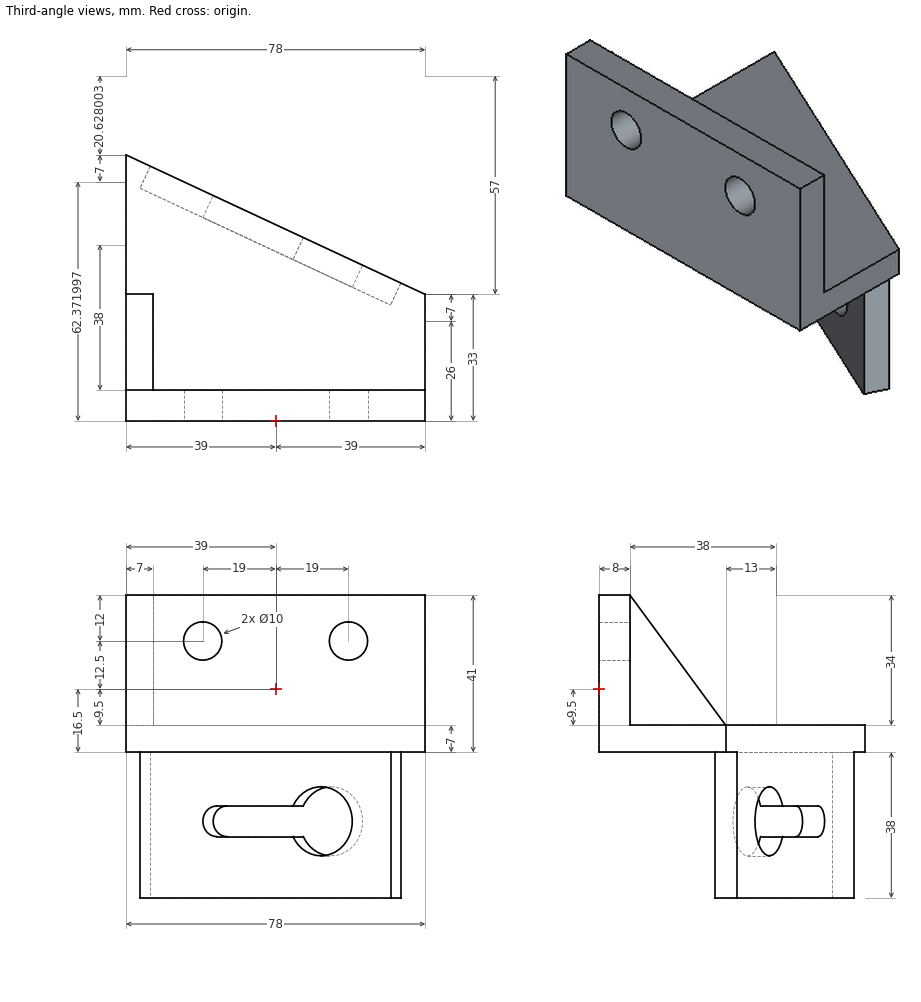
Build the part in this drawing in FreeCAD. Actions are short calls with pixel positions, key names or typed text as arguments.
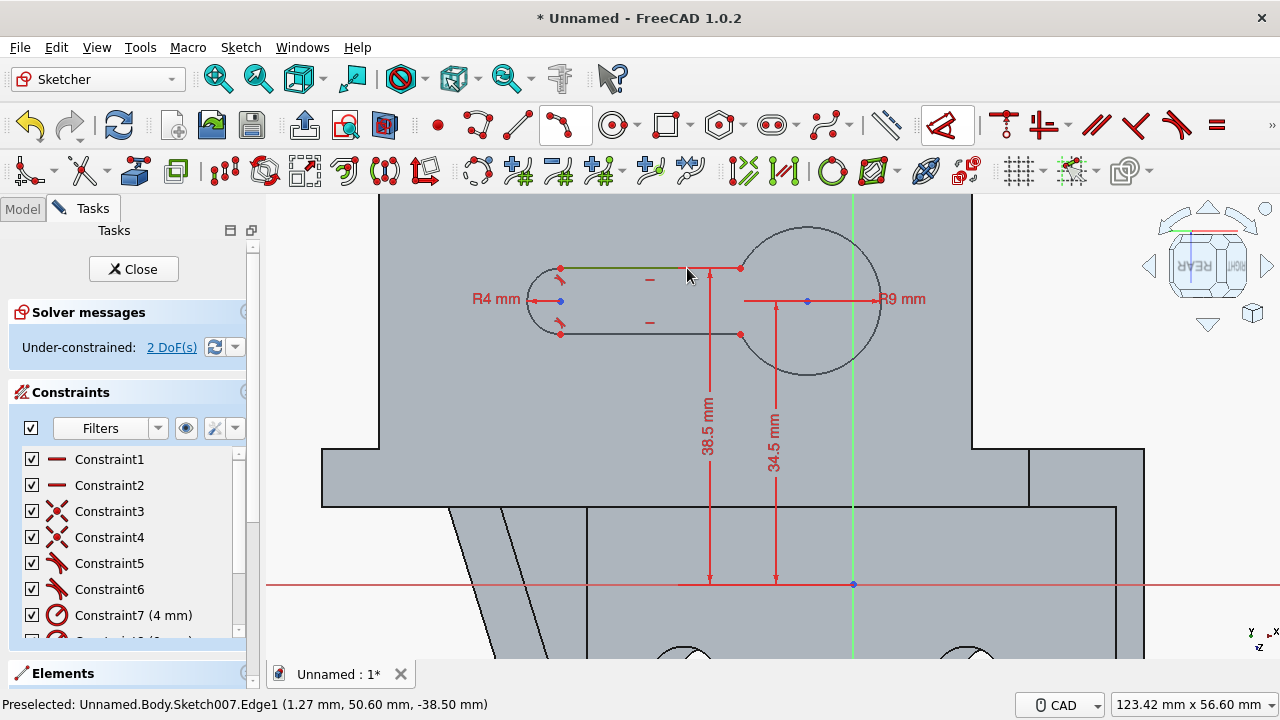
key(l)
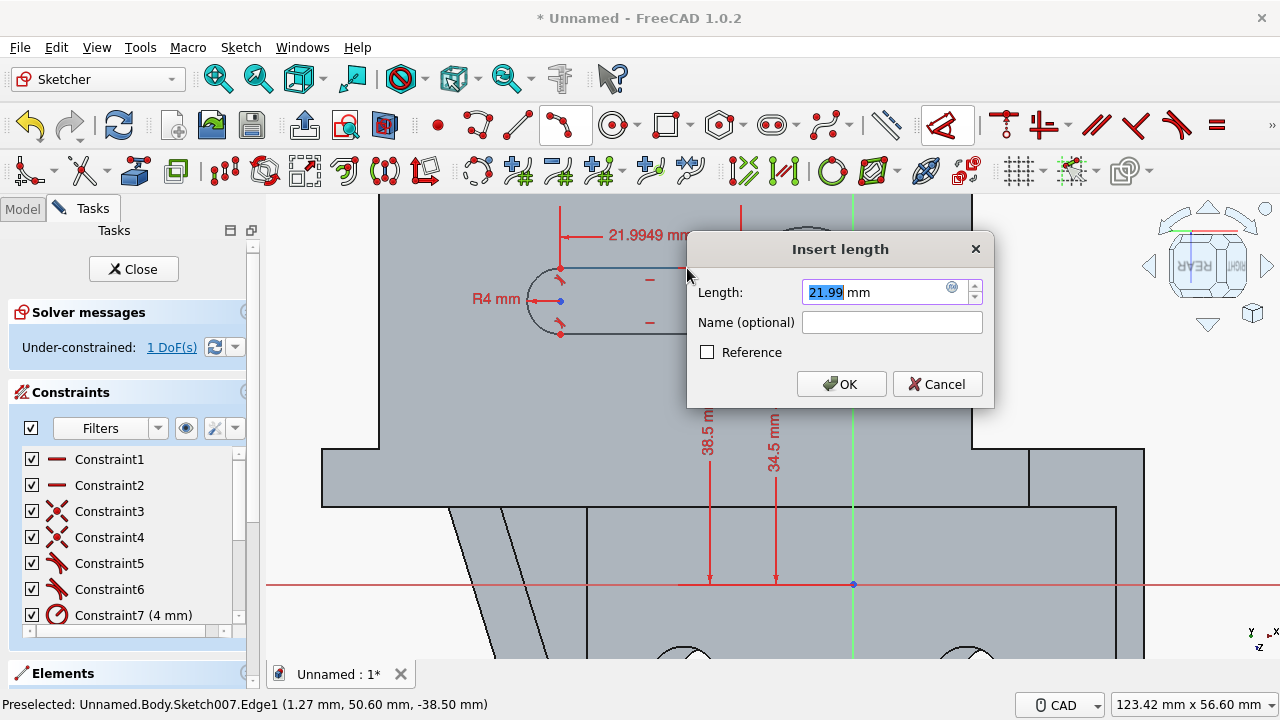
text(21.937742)
key(Return)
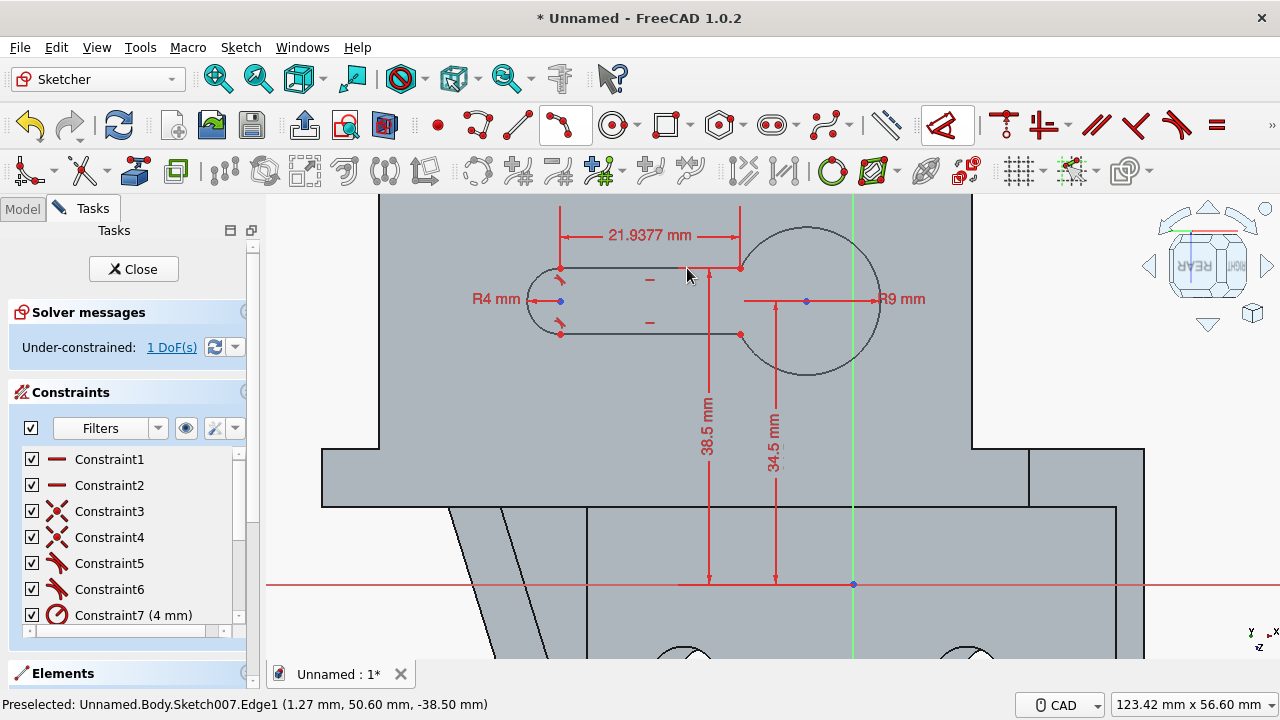
click(807, 301)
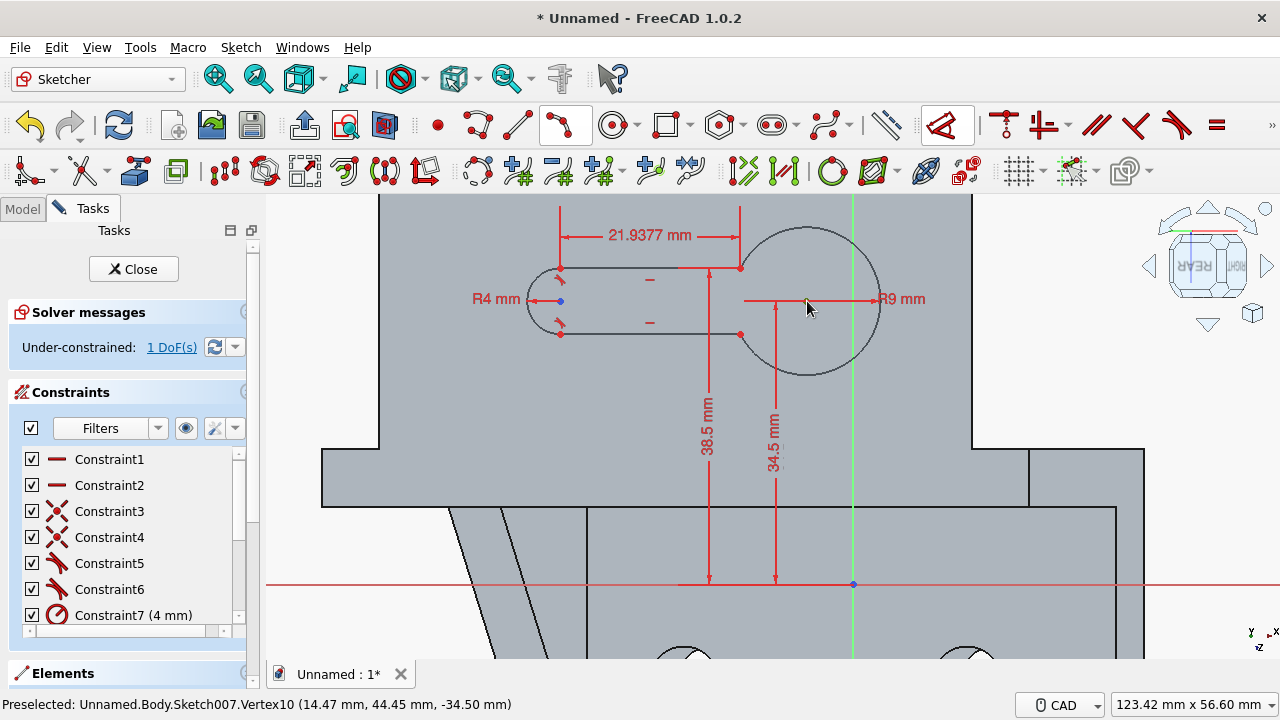
key(l)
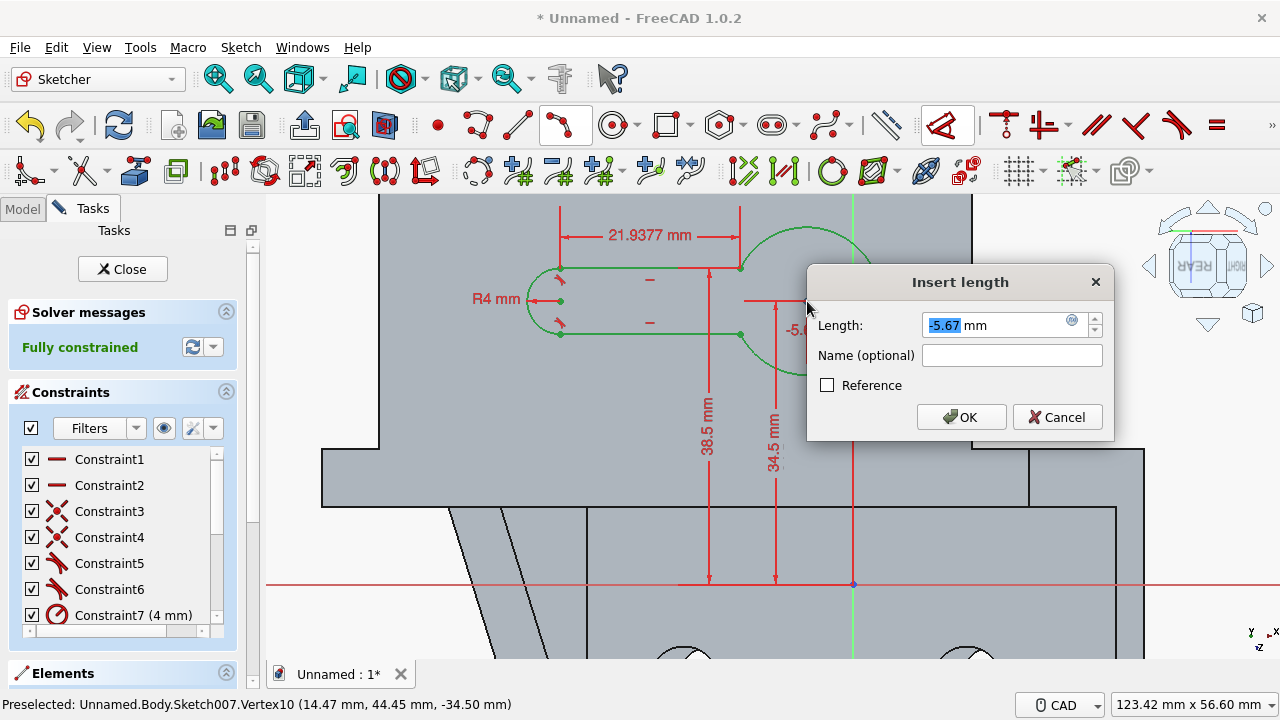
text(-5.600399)
key(Return)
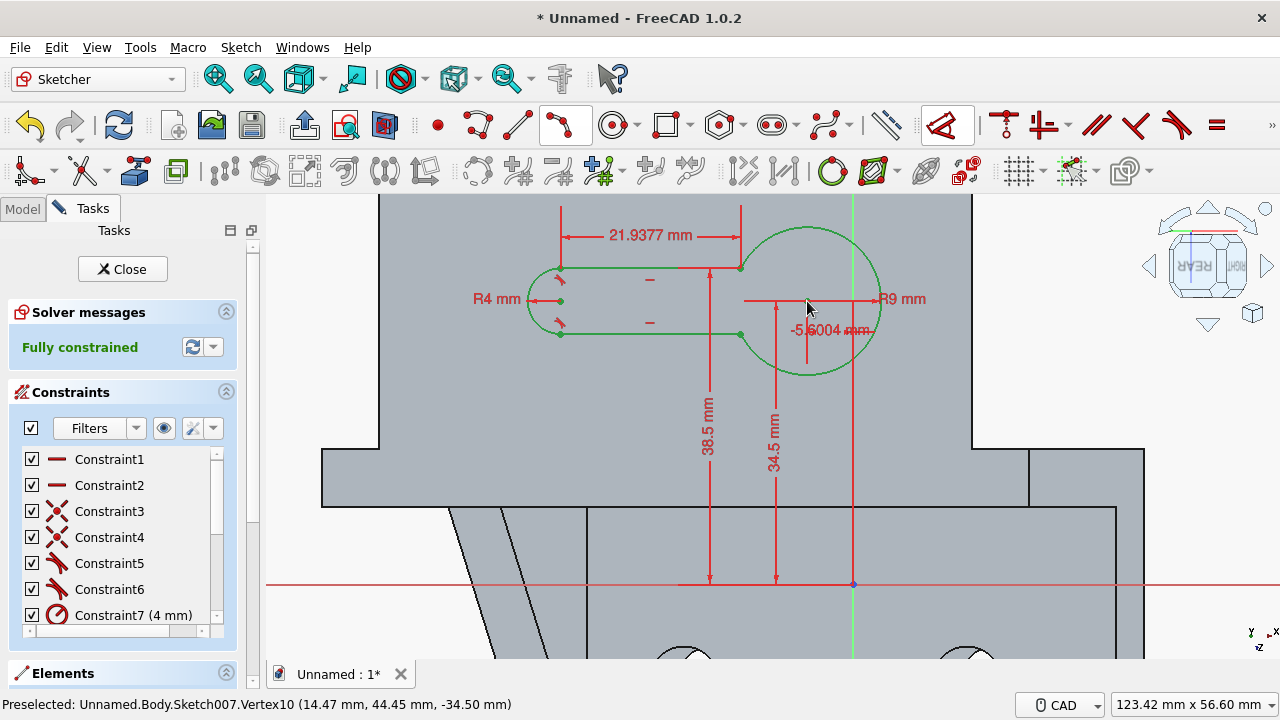
click(123, 269)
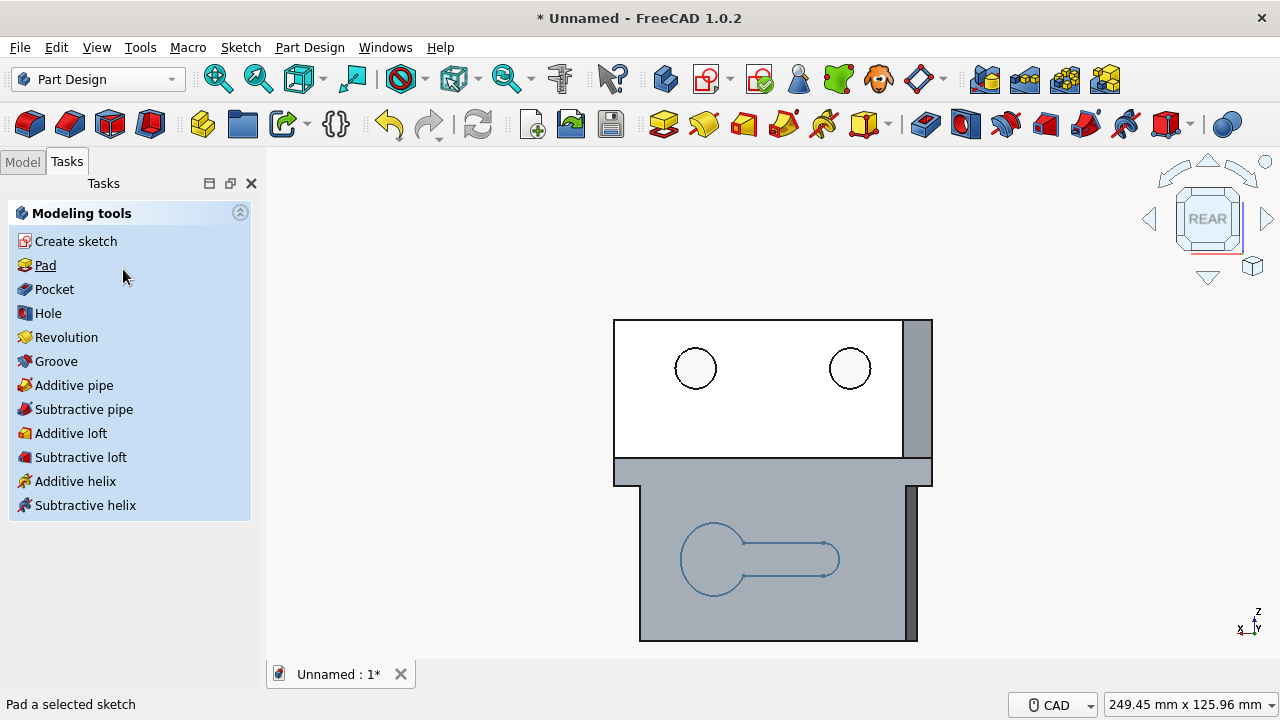
click(926, 124)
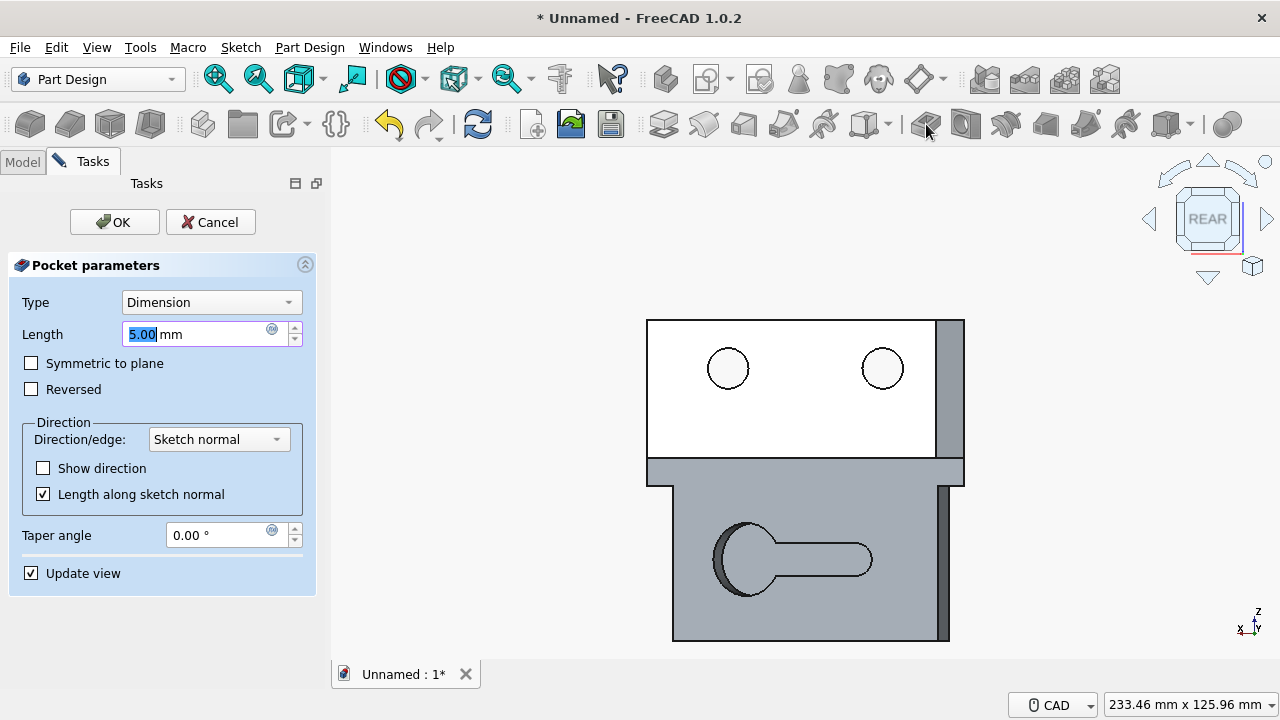
click(212, 302)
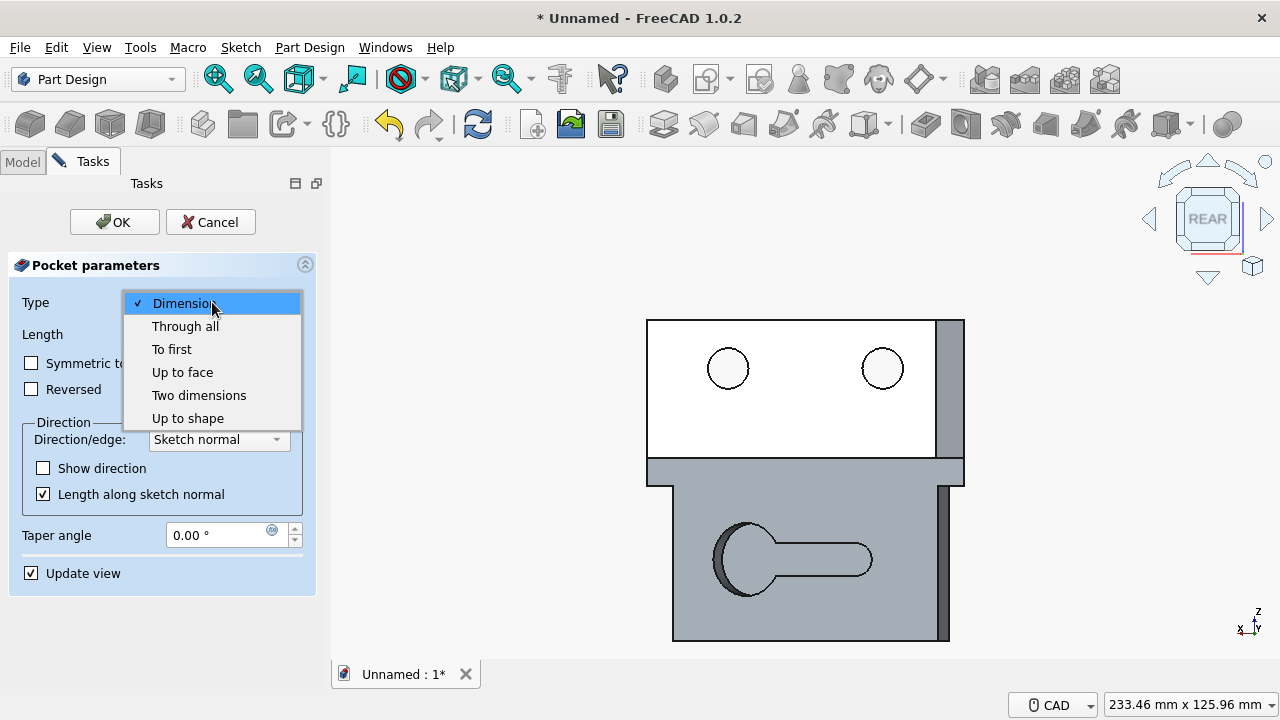
click(212, 350)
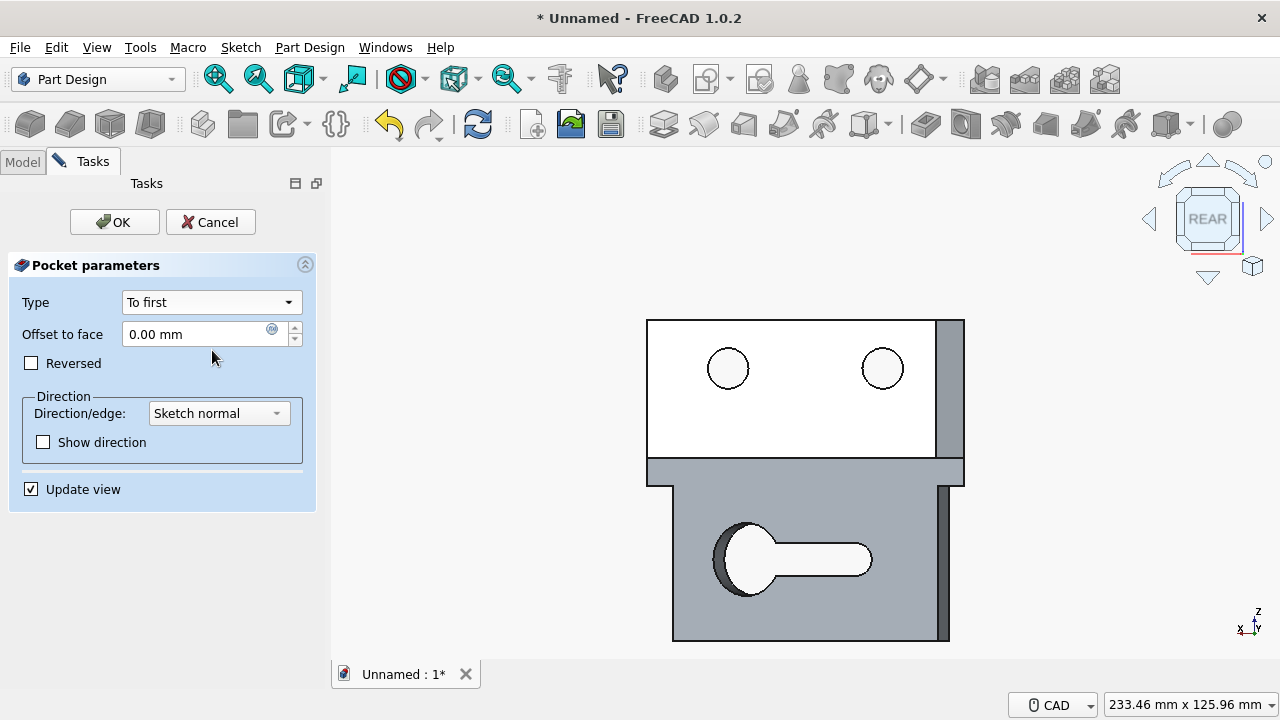
click(115, 222)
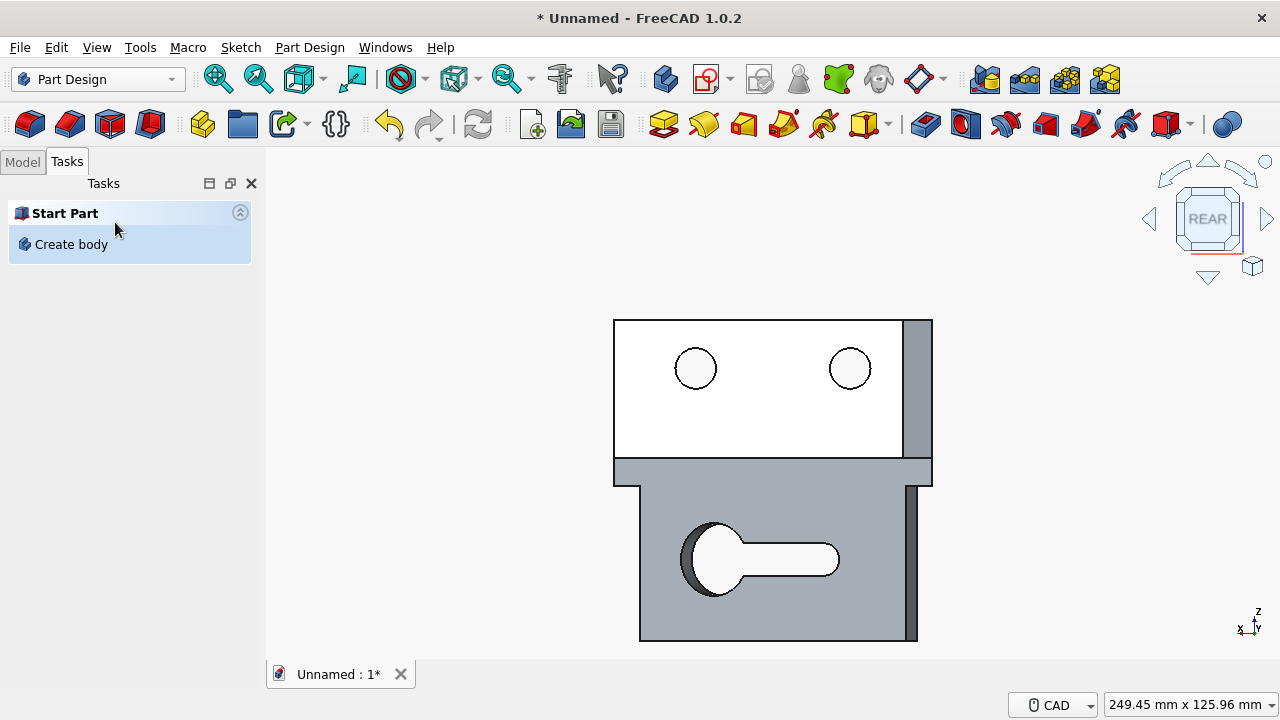
key(0)